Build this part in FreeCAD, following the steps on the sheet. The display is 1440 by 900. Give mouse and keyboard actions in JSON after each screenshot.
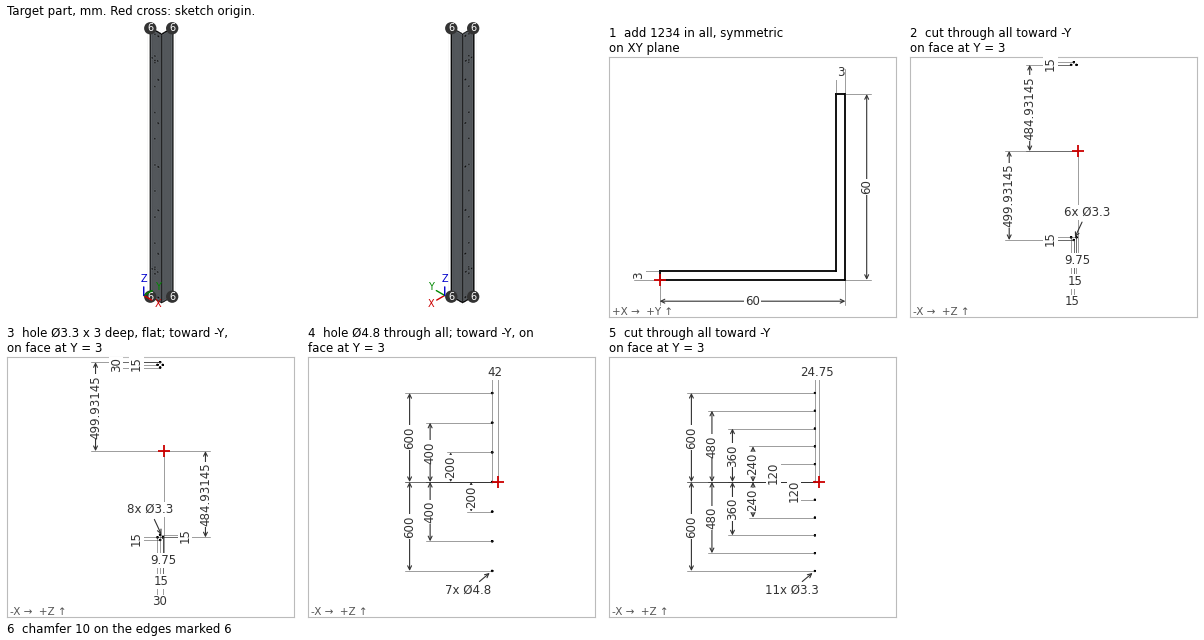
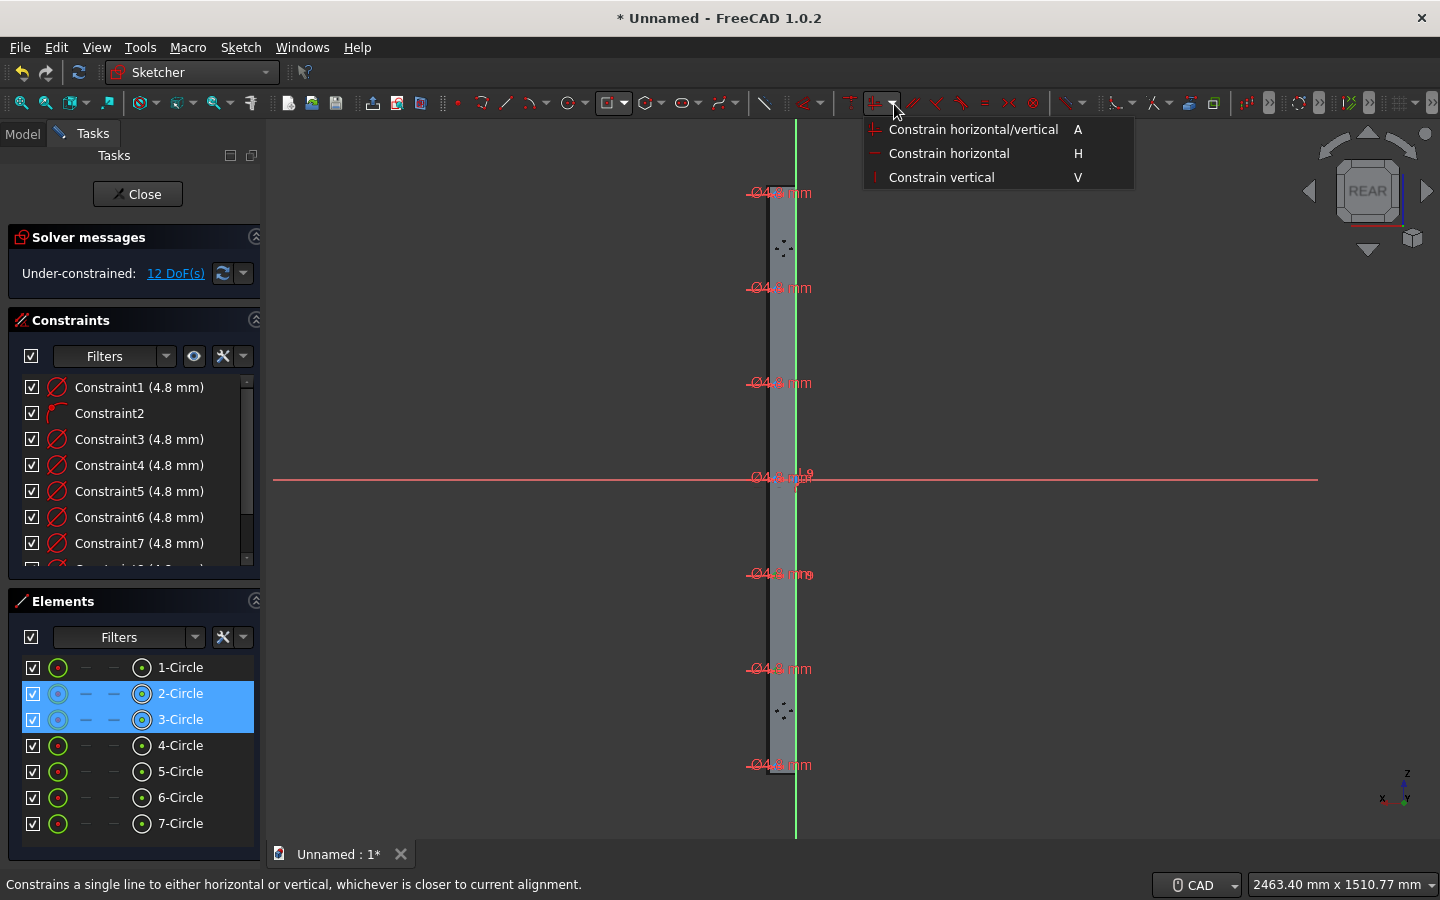
{"action": "left_click", "coordinate": [999, 177]}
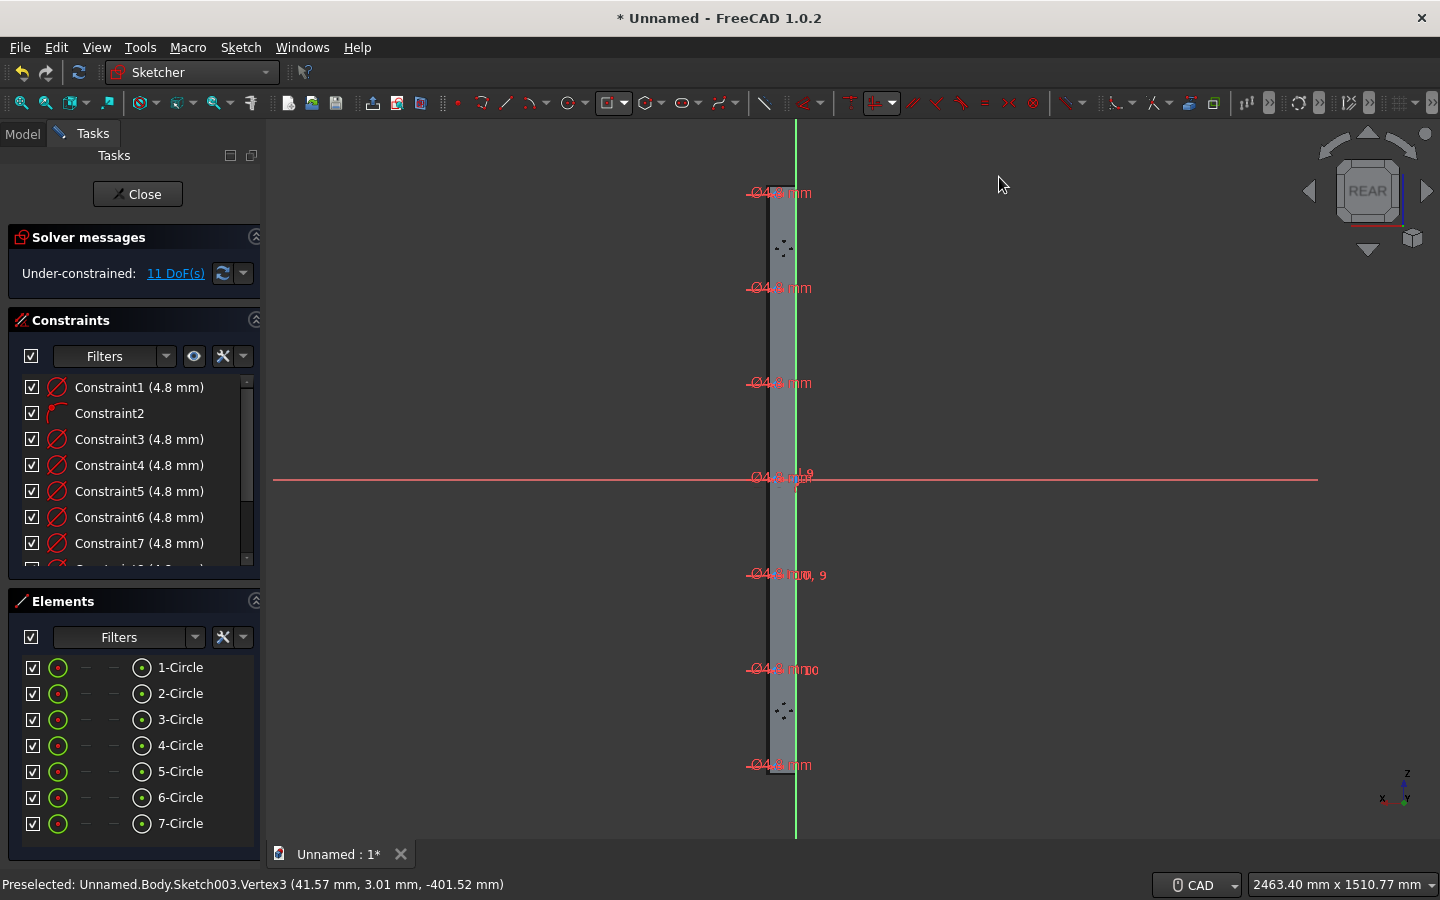
{"action": "left_click", "coordinate": [776, 671]}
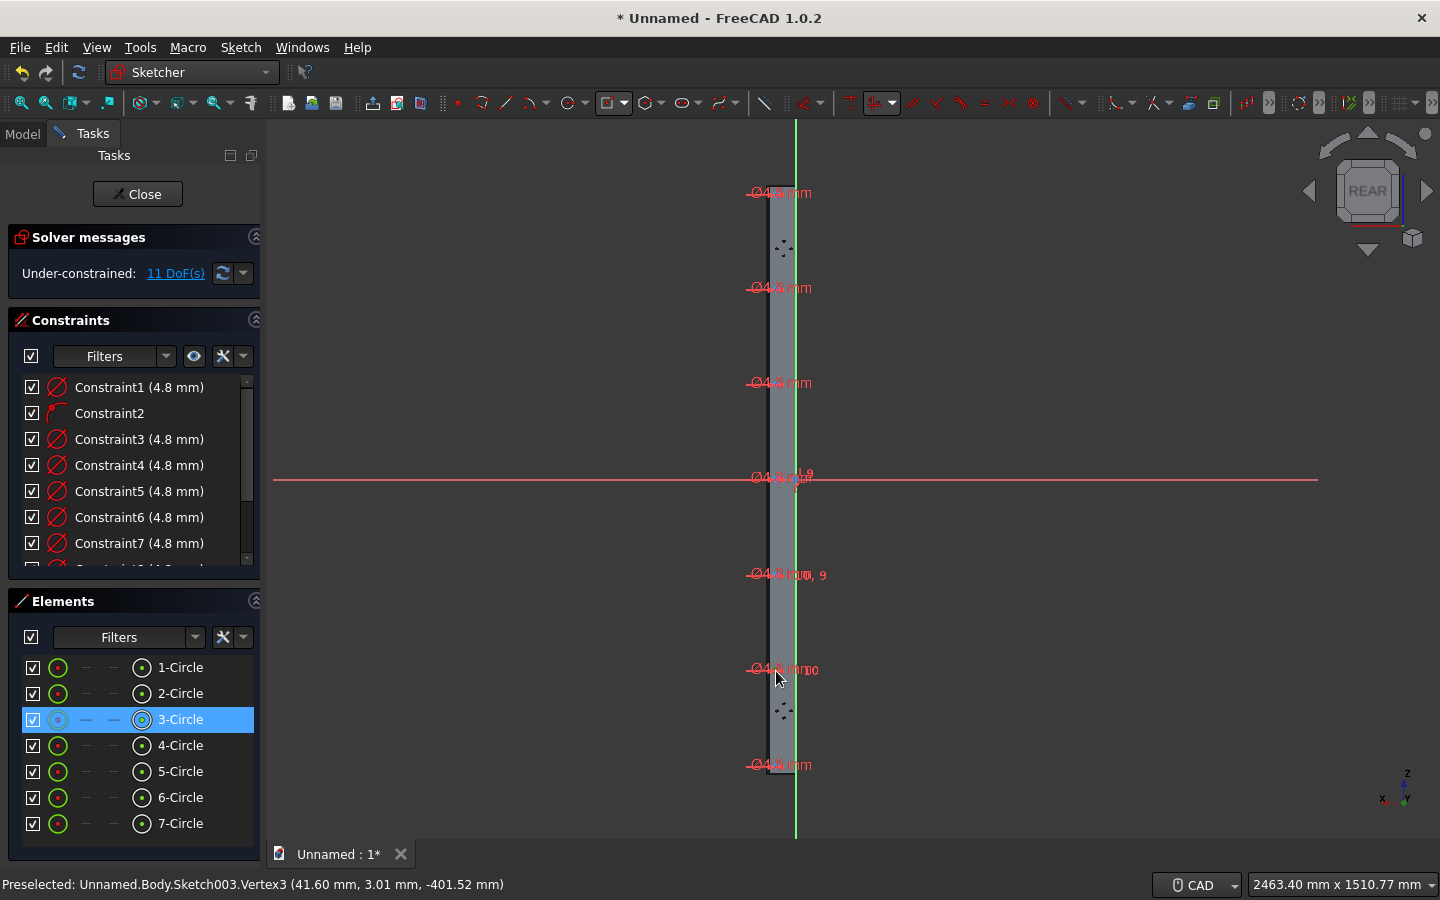
{"action": "left_click", "coordinate": [776, 767]}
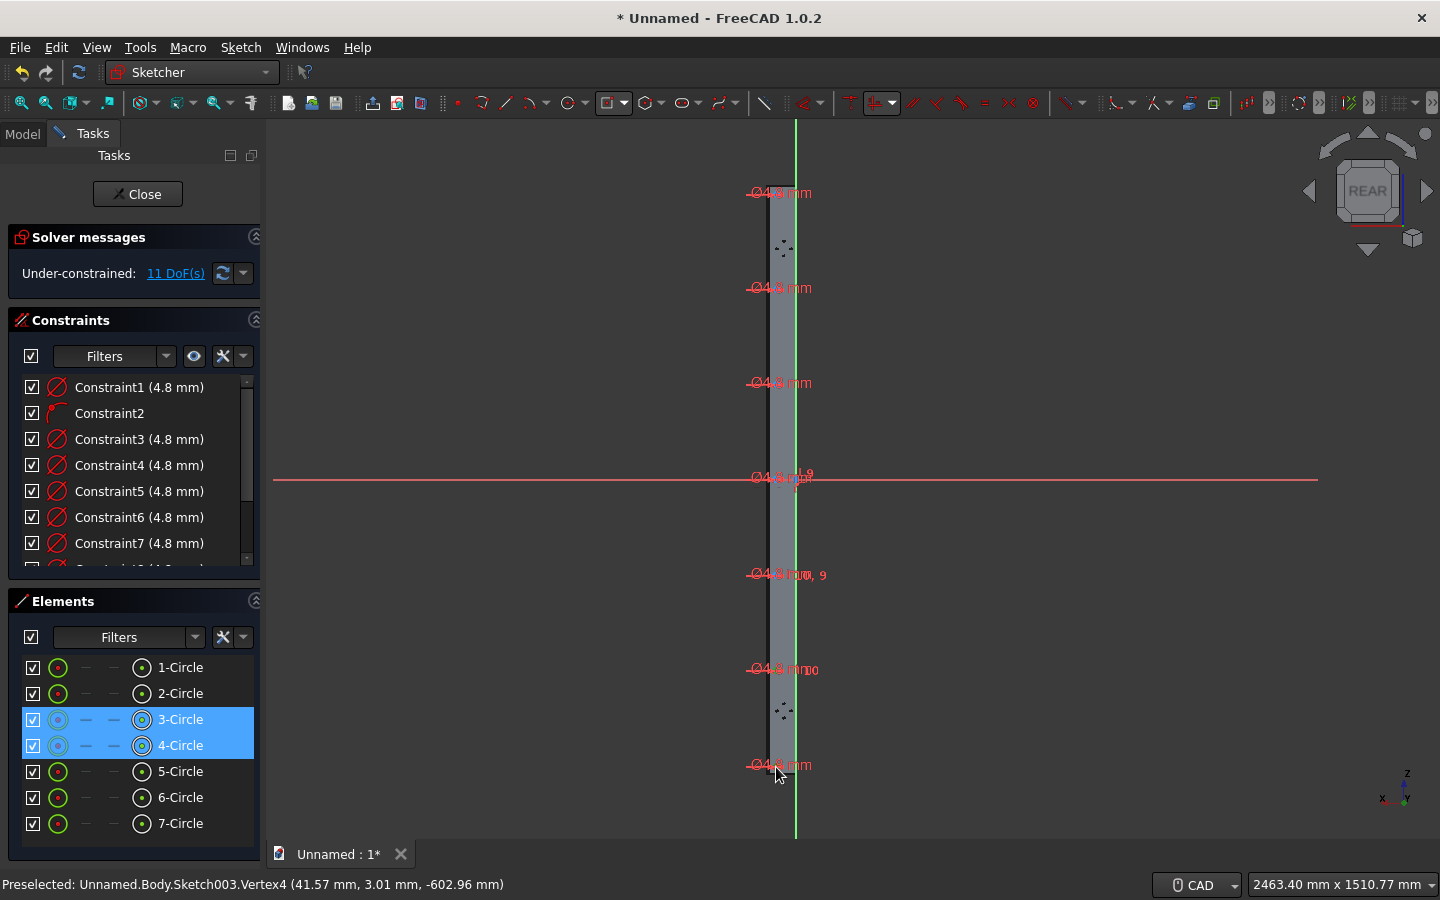
{"action": "left_click", "coordinate": [894, 104]}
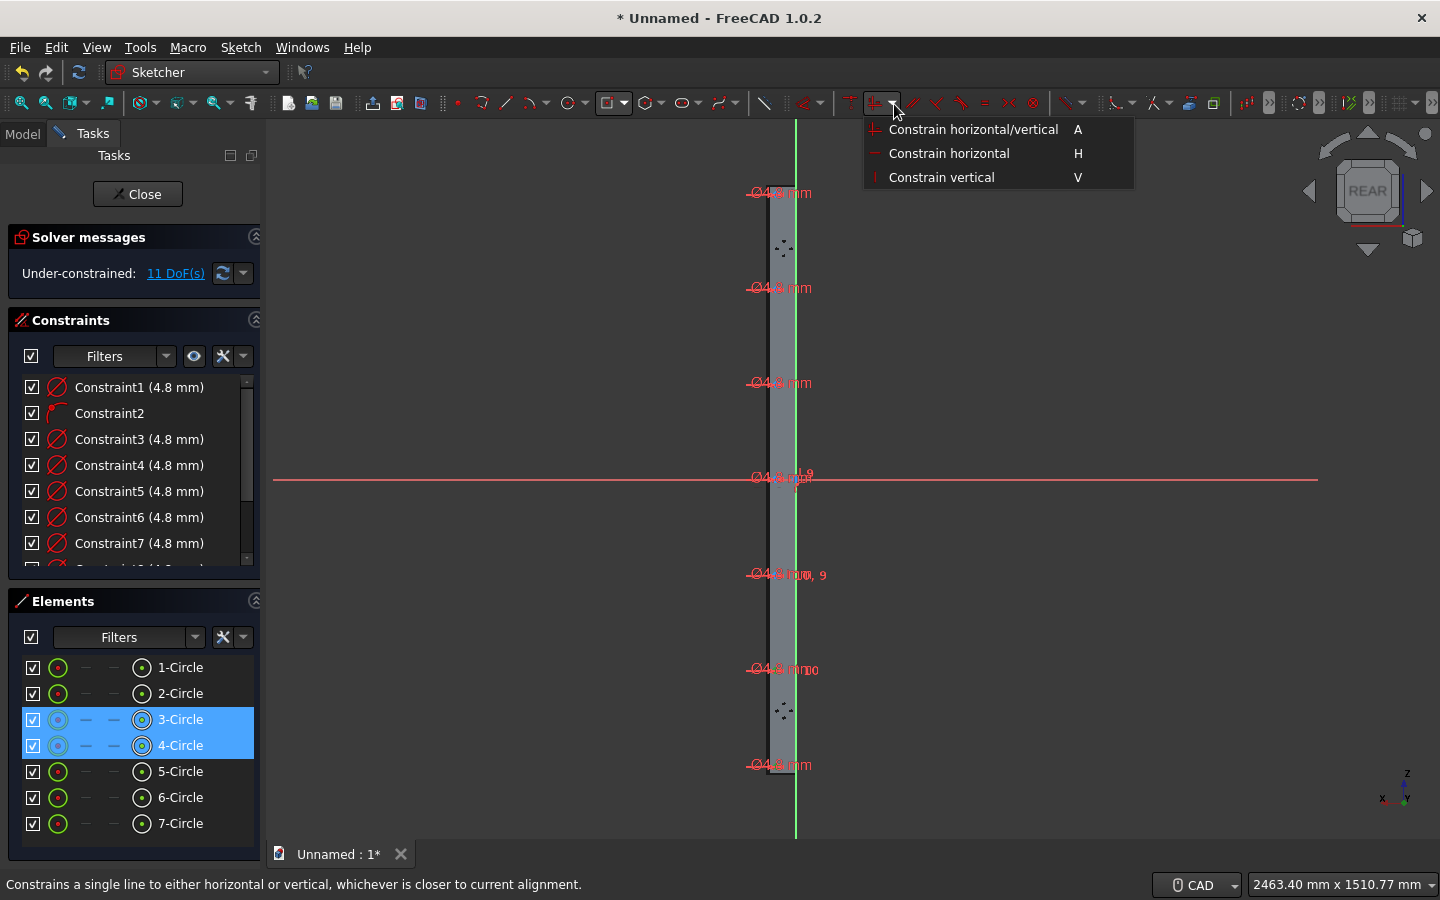
{"action": "left_click", "coordinate": [999, 177]}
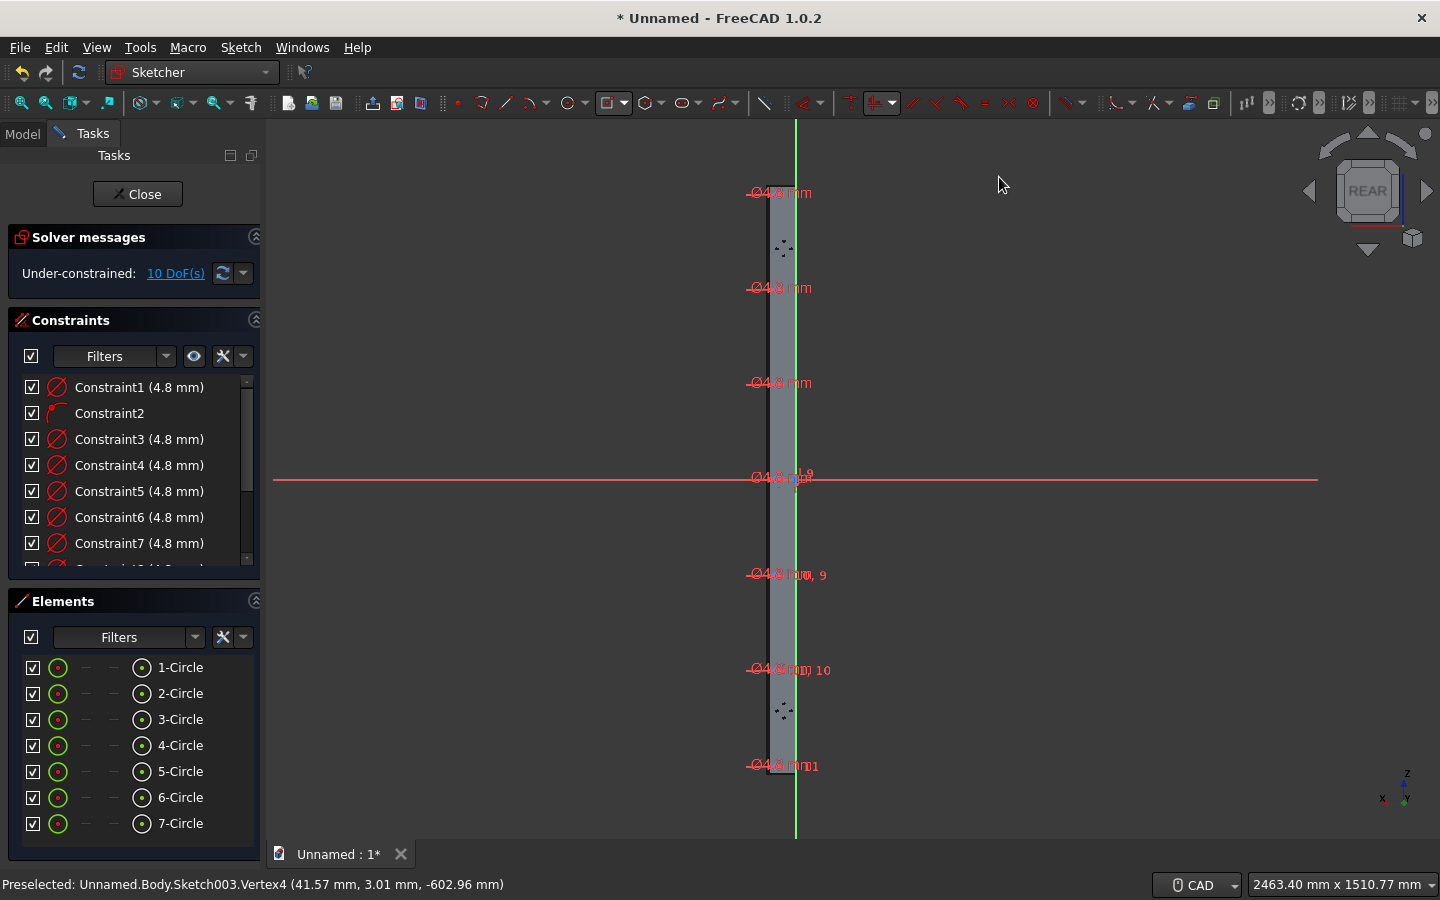
{"action": "left_click", "coordinate": [776, 480]}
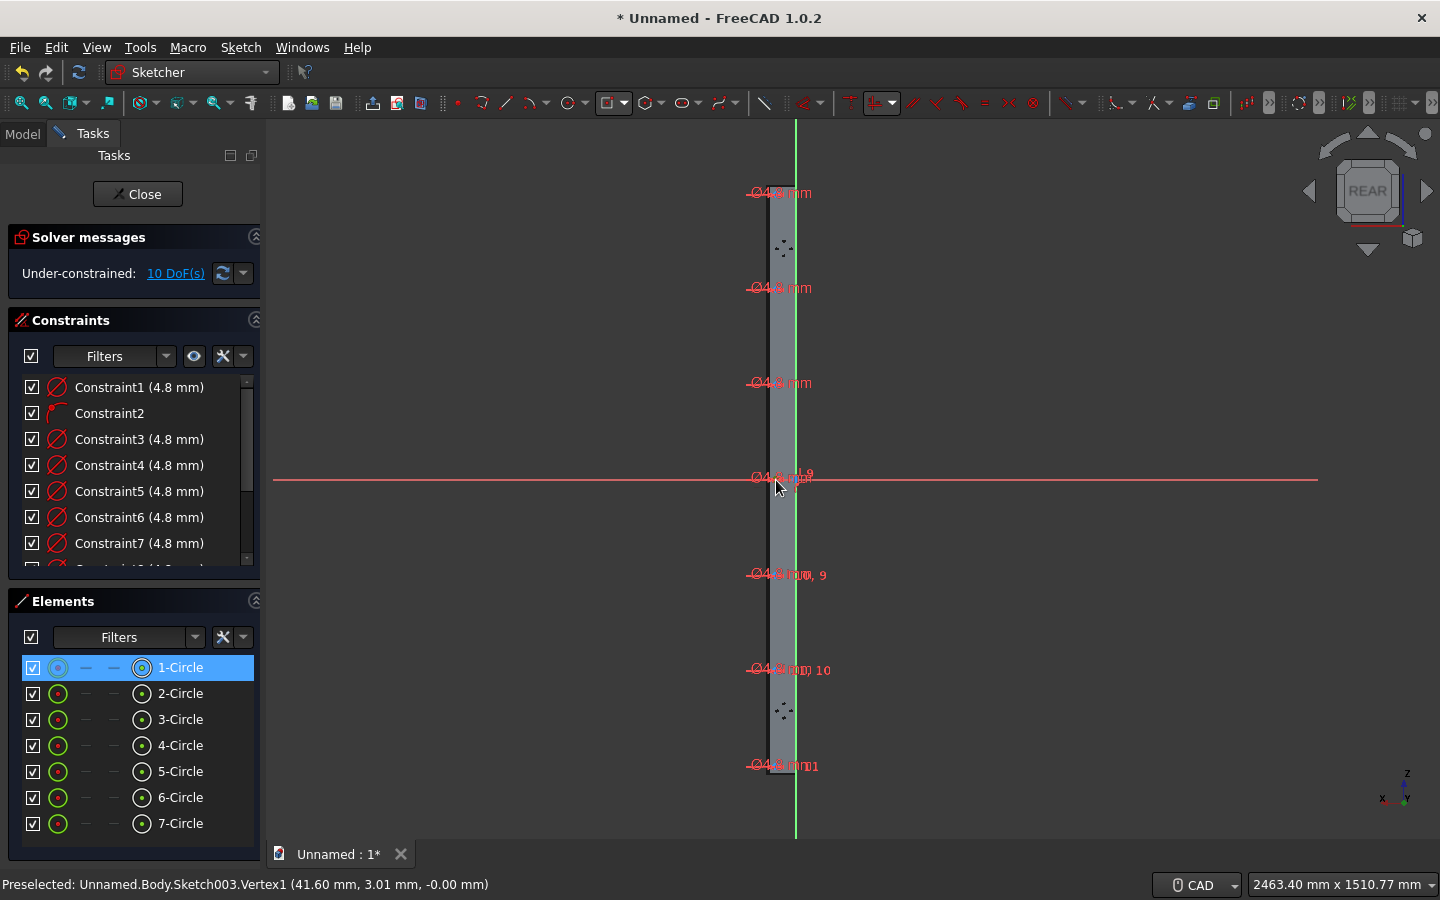
{"action": "left_click", "coordinate": [776, 195]}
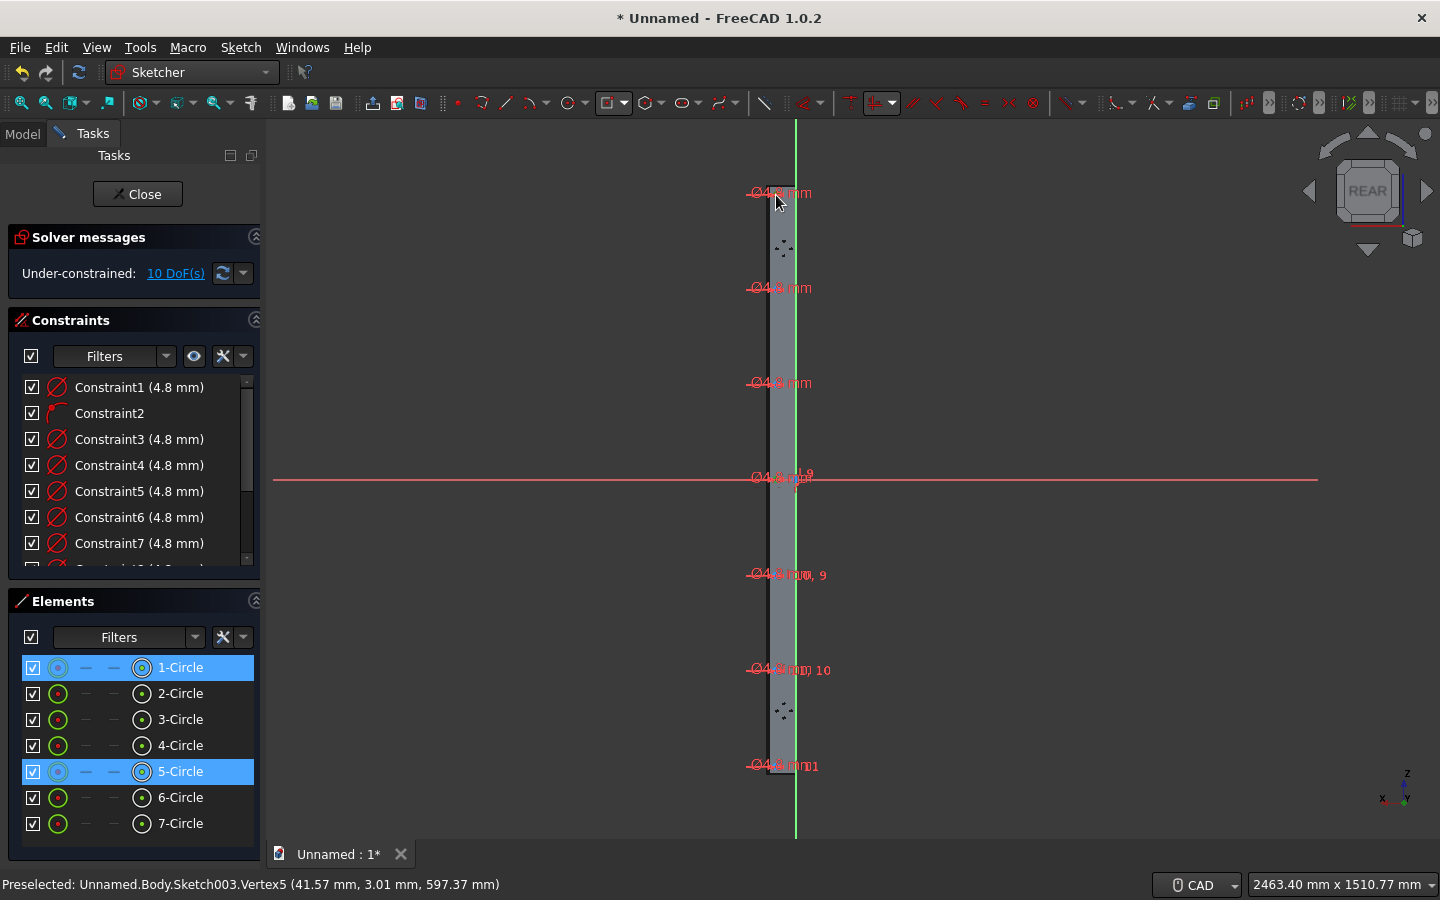
{"action": "left_click", "coordinate": [894, 104]}